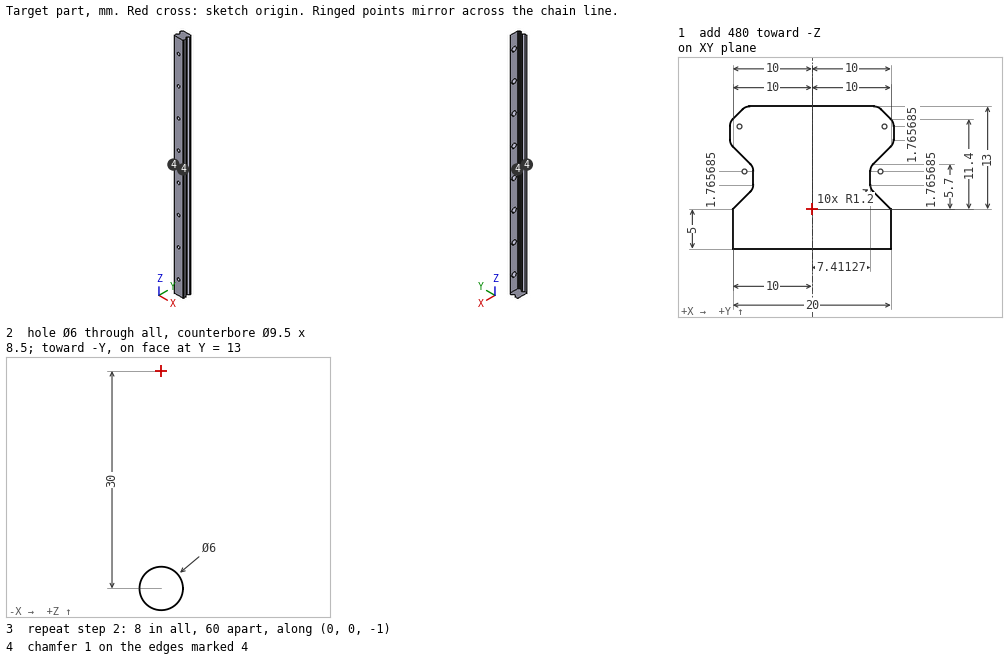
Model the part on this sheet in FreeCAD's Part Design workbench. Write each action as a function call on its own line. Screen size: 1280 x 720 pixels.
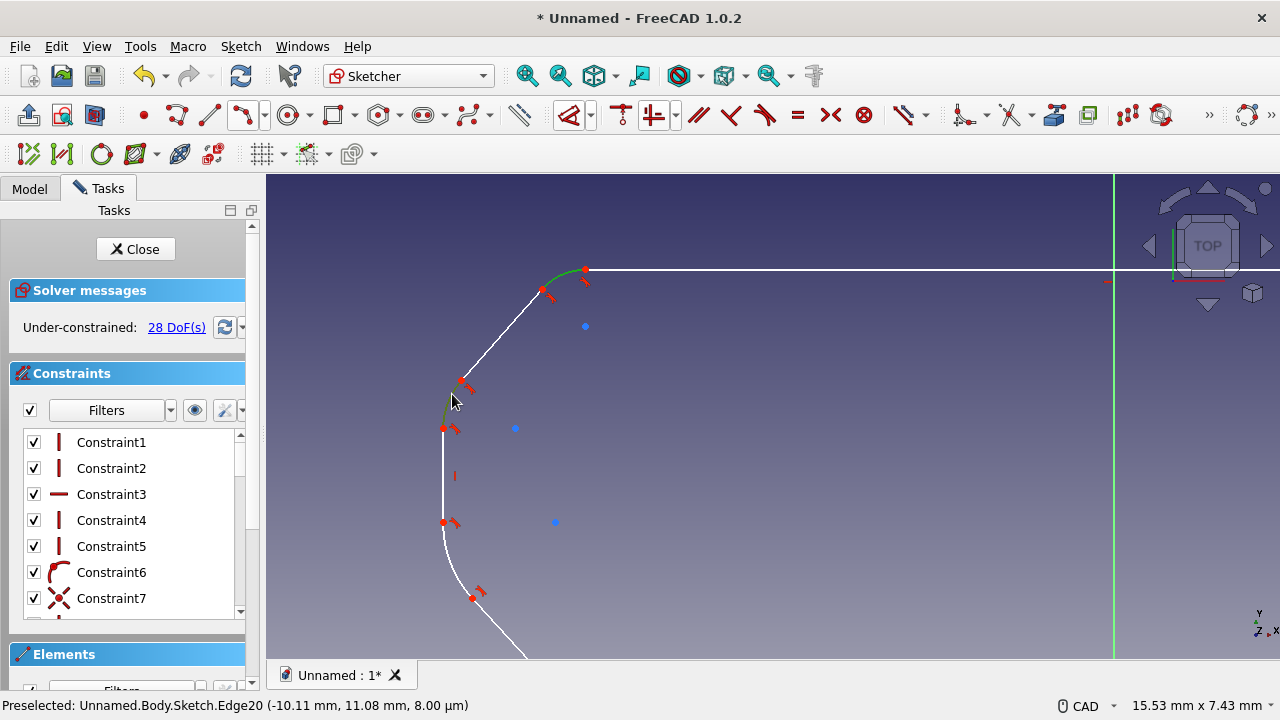
click(446, 548)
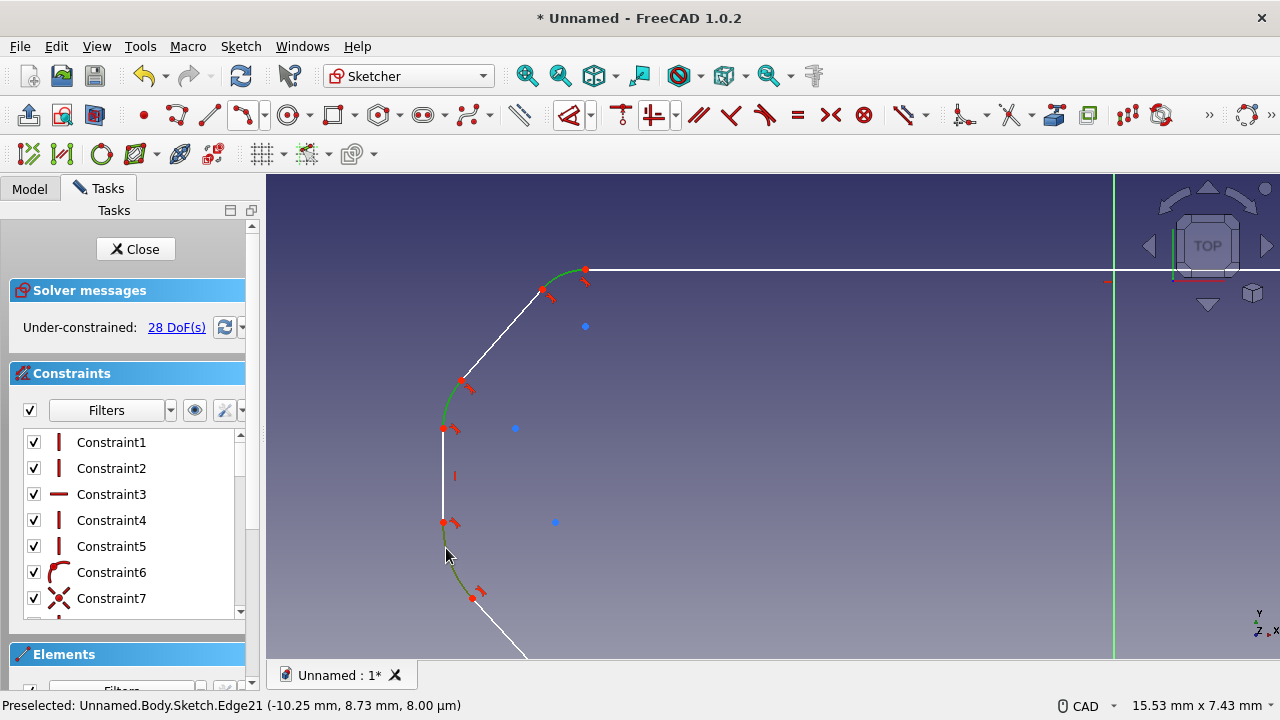
scroll(570, 274, down, 7)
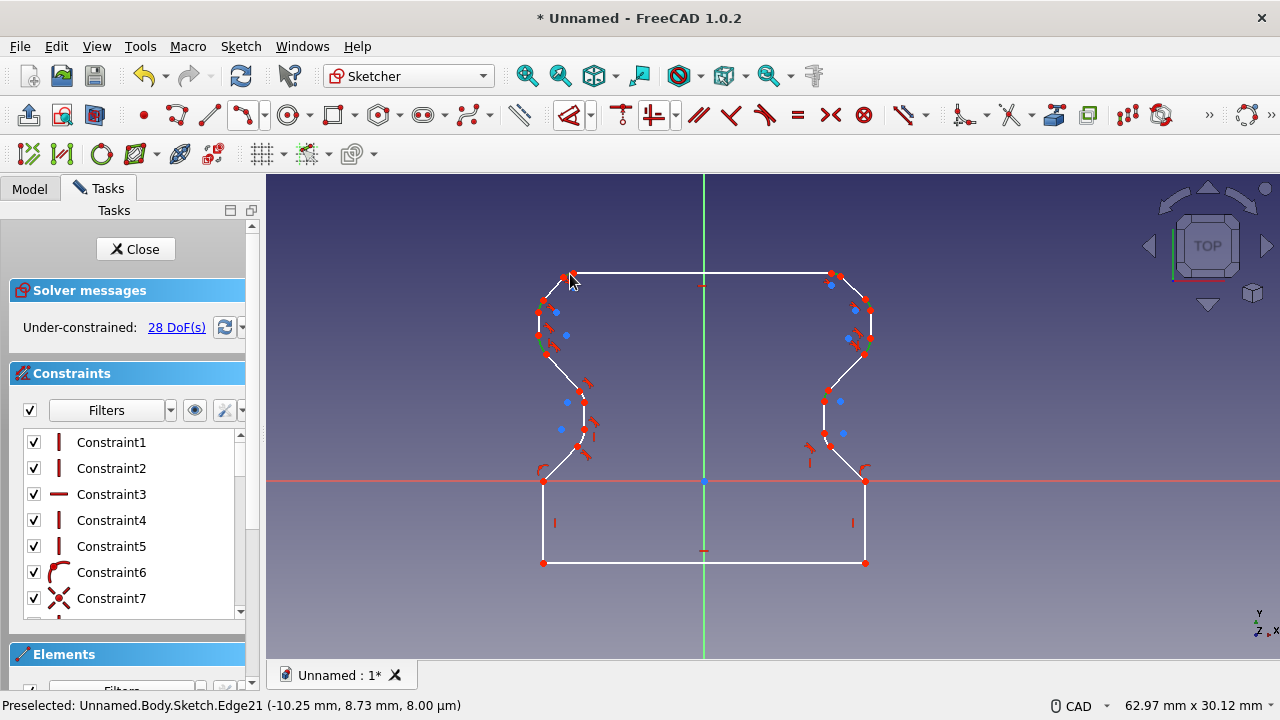
scroll(584, 399, up, 7)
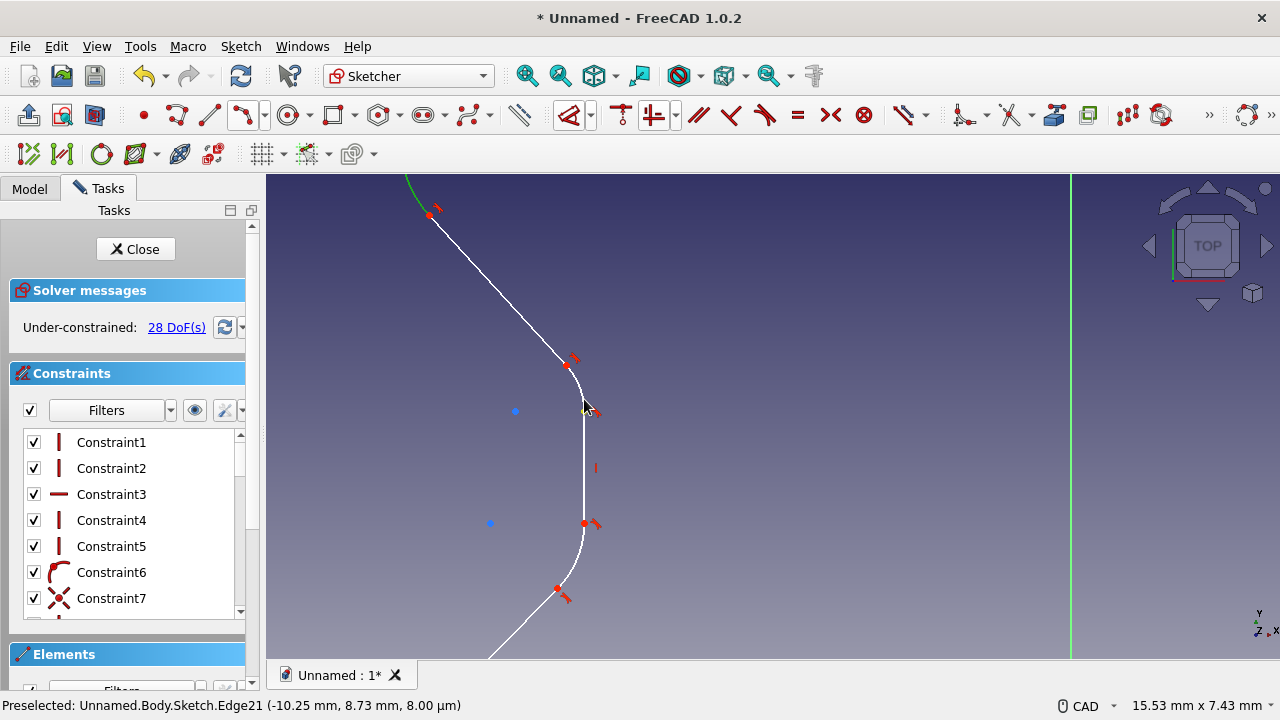
click(583, 397)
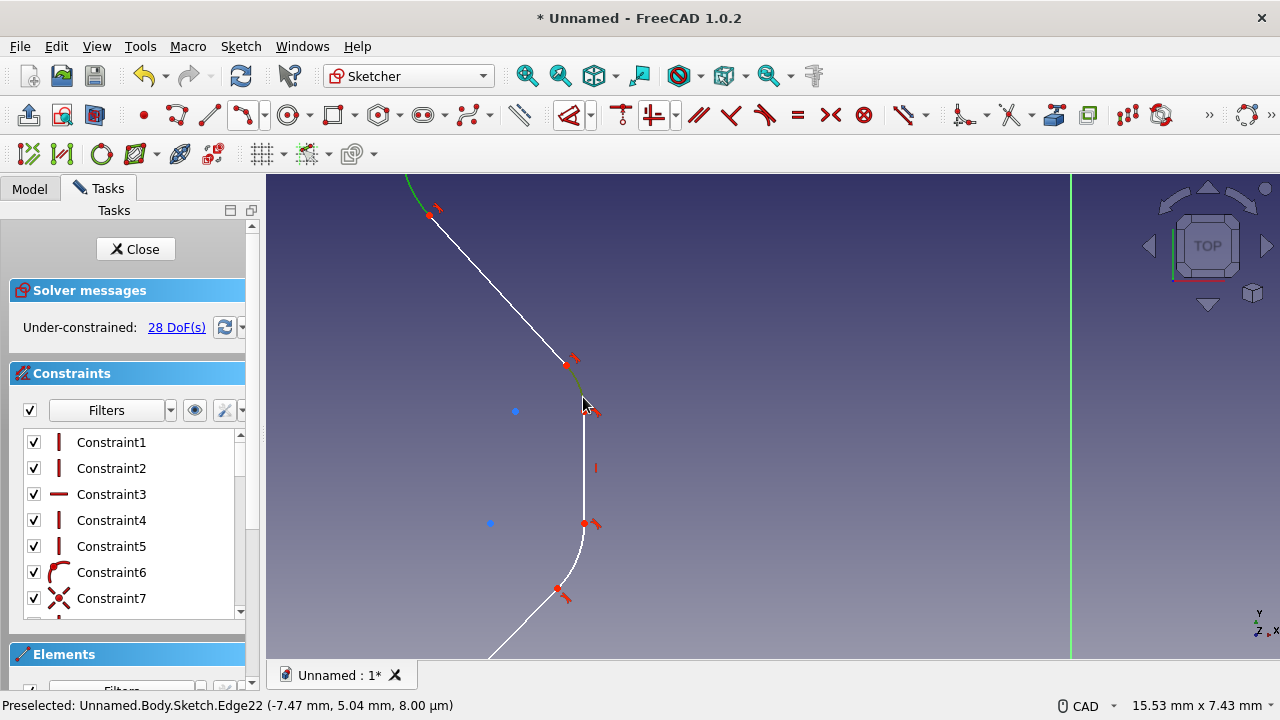
click(571, 572)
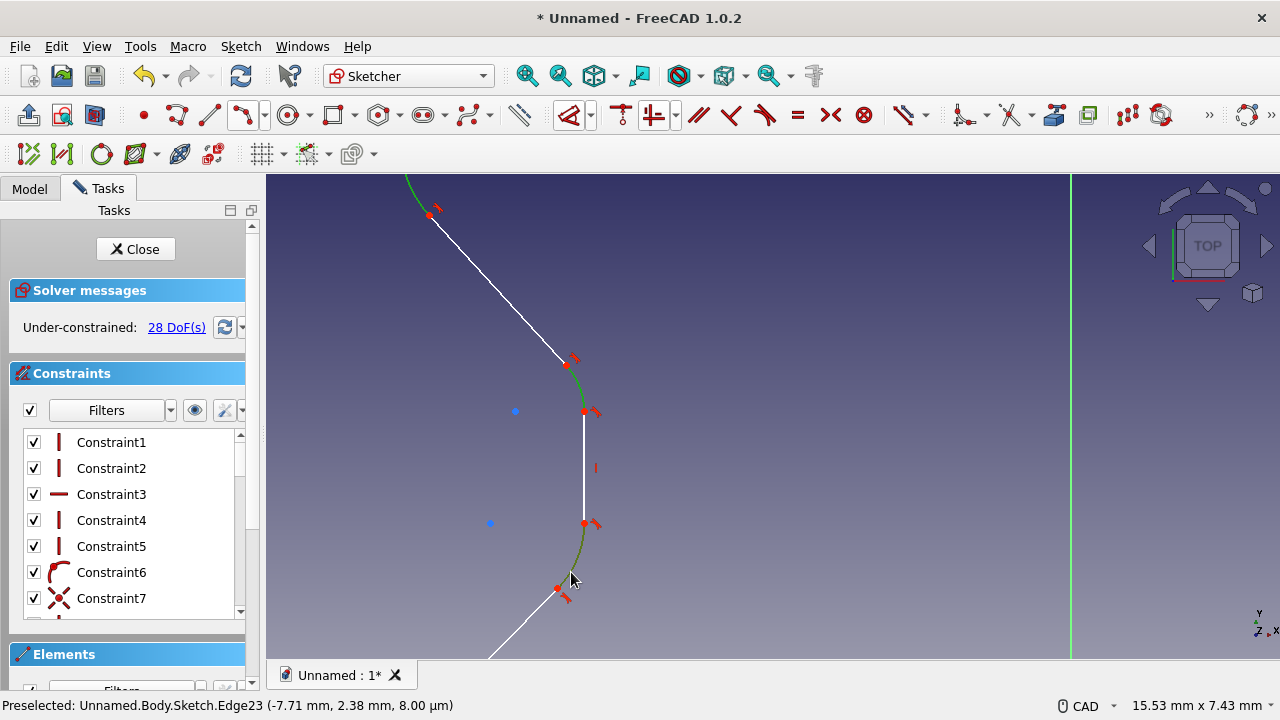
scroll(584, 399, down, 7)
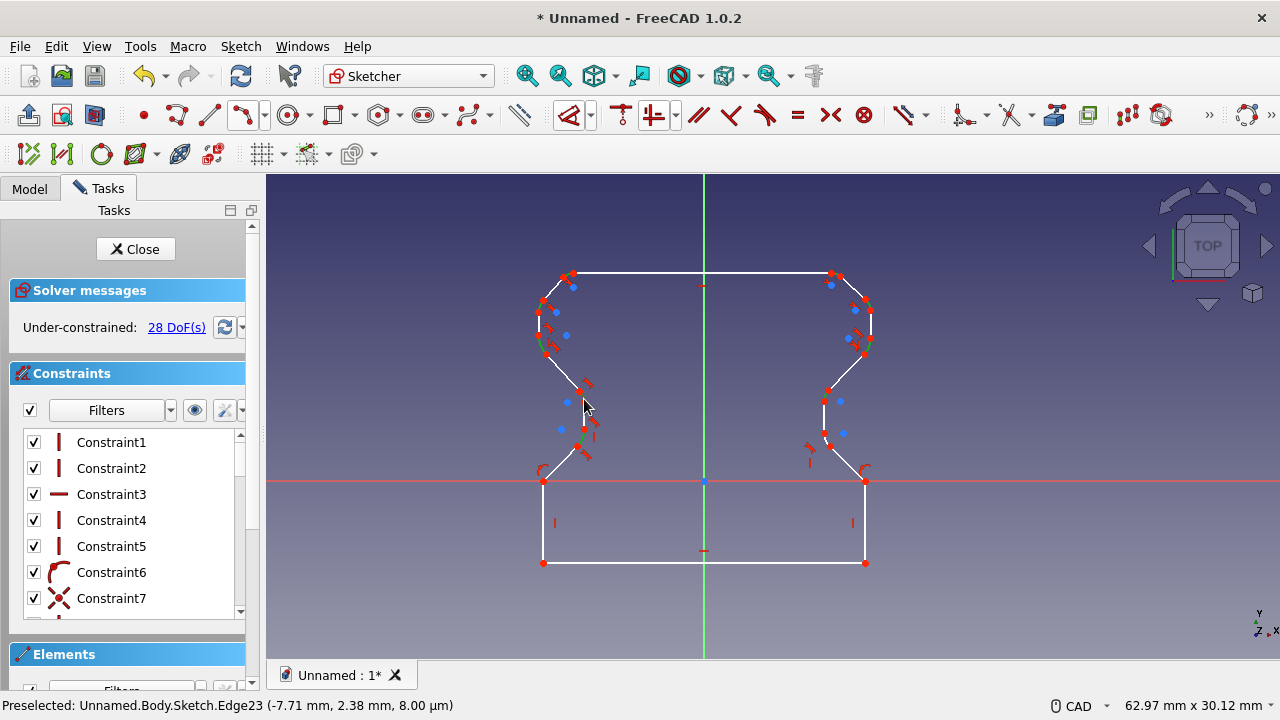
scroll(825, 438, up, 6)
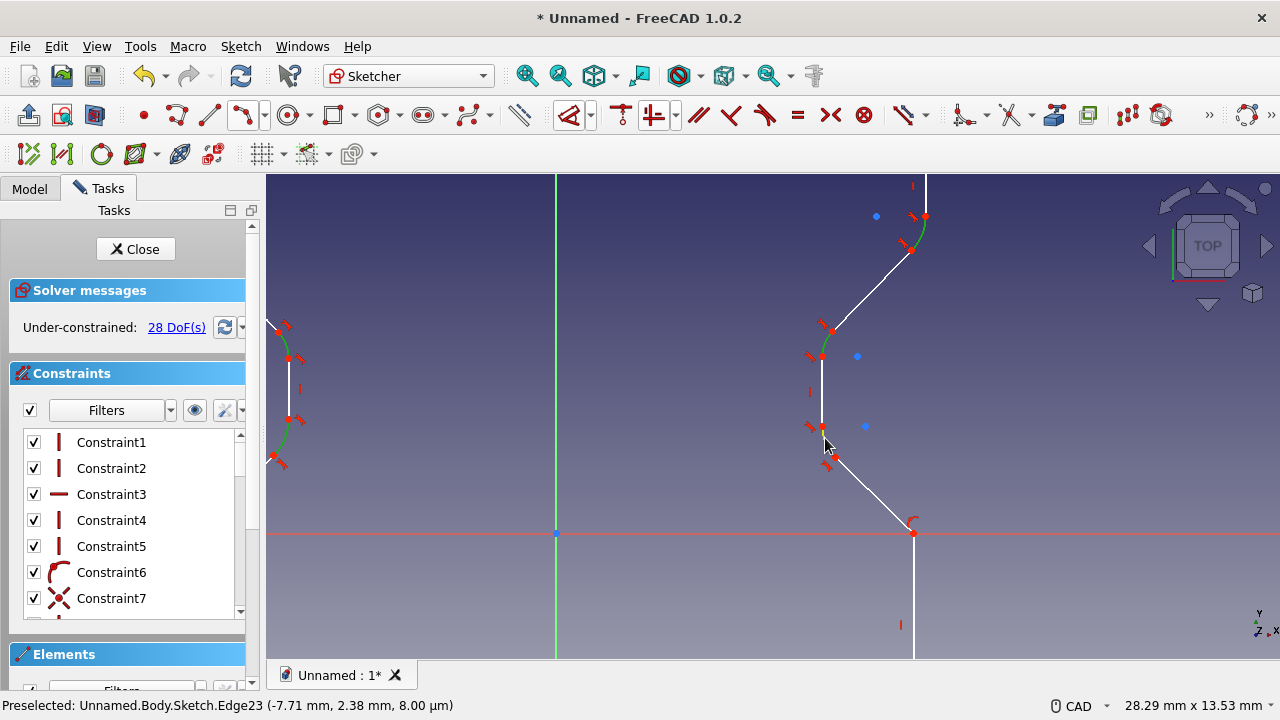
click(823, 436)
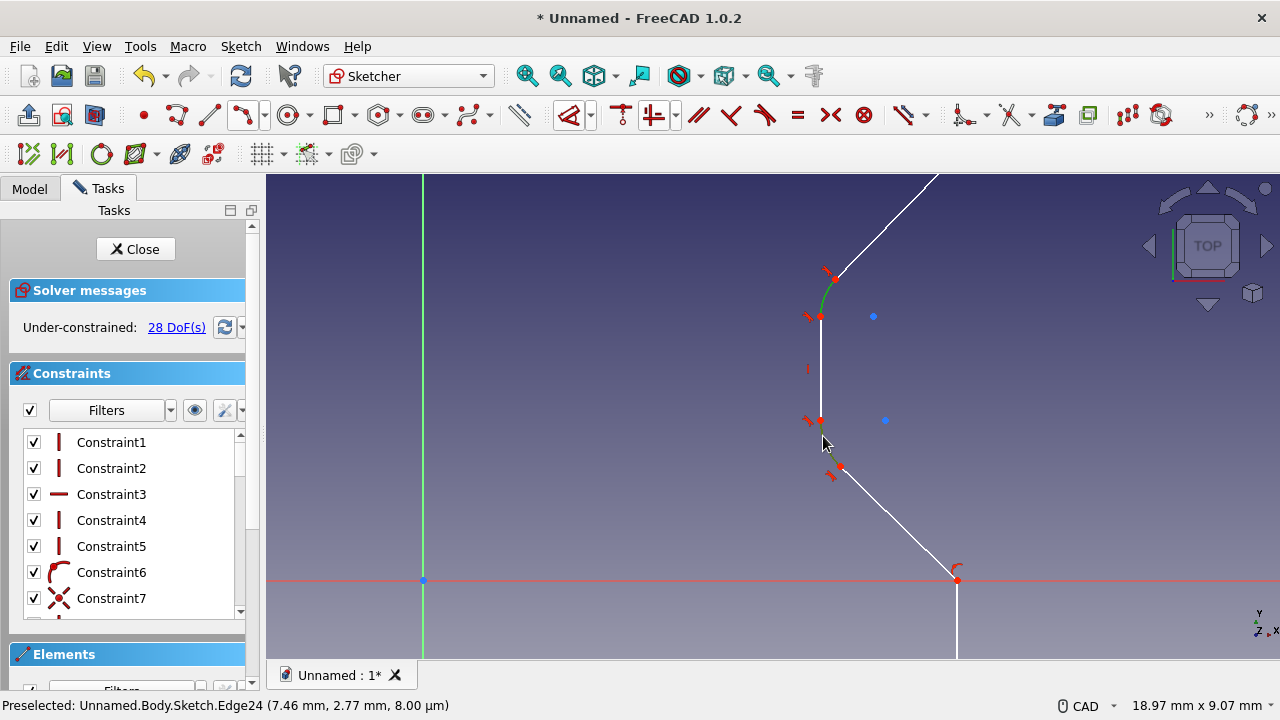
key(e)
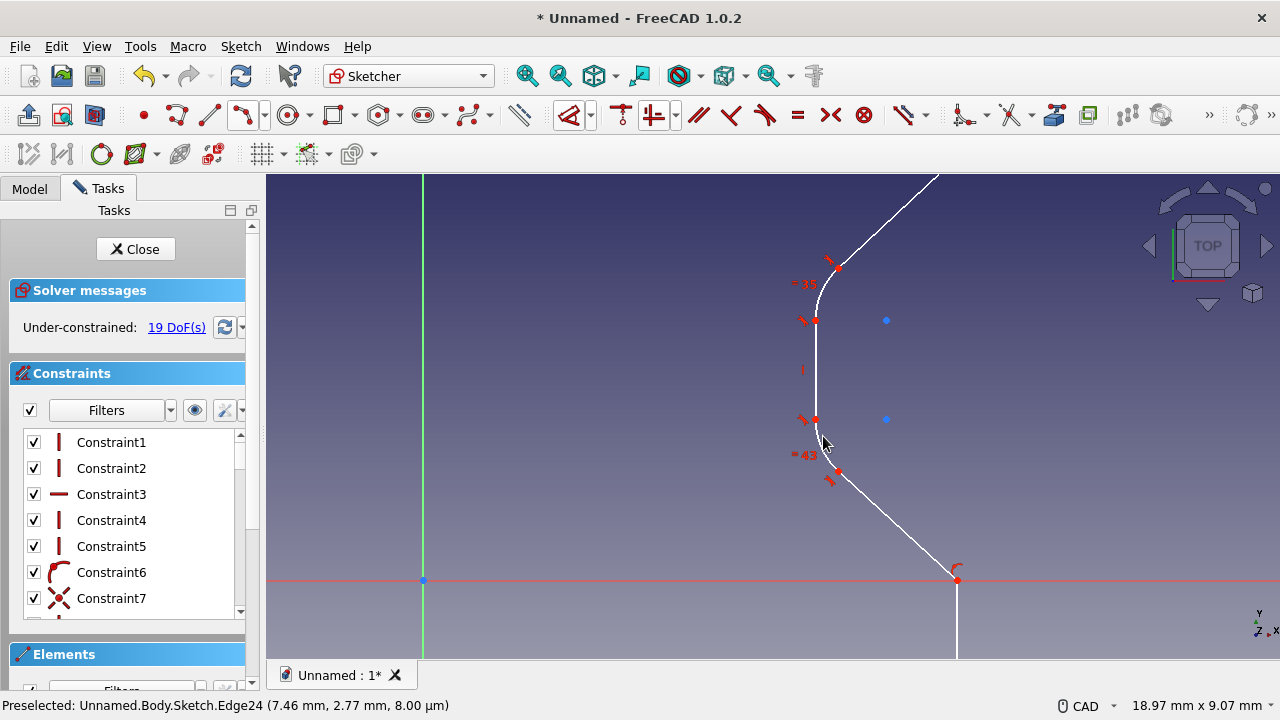
scroll(826, 438, down, 6)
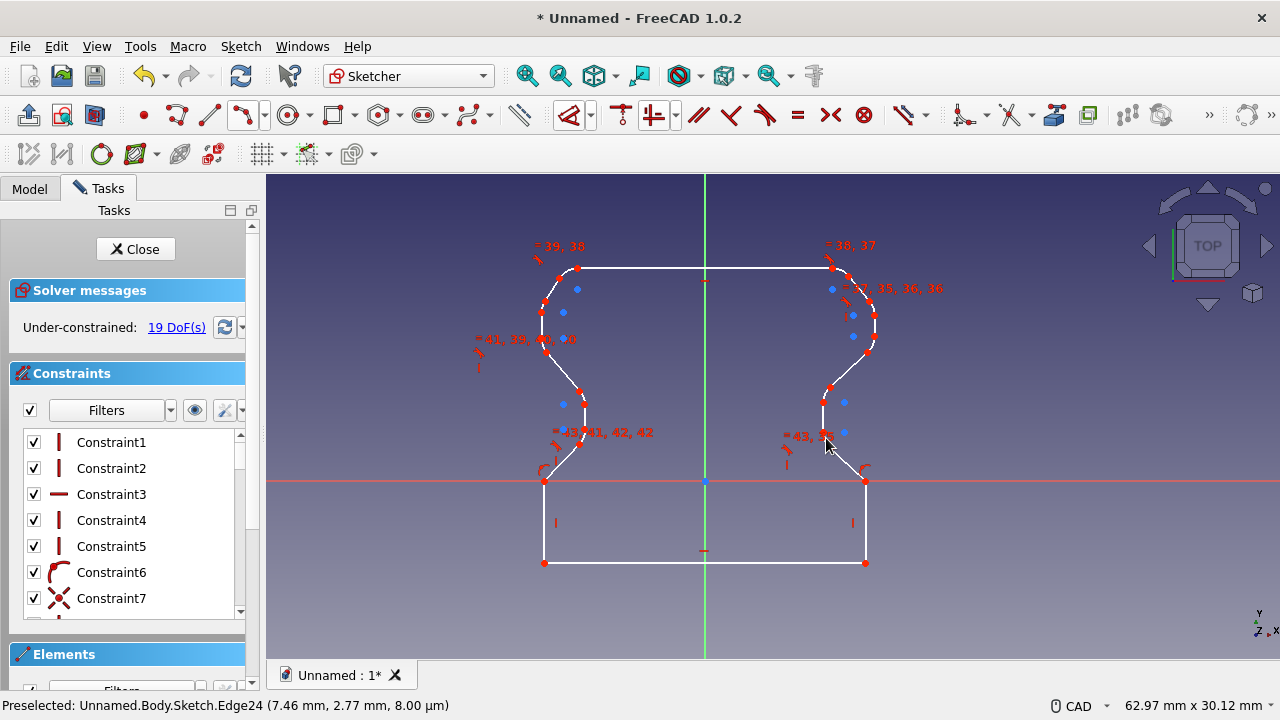
click(853, 315)